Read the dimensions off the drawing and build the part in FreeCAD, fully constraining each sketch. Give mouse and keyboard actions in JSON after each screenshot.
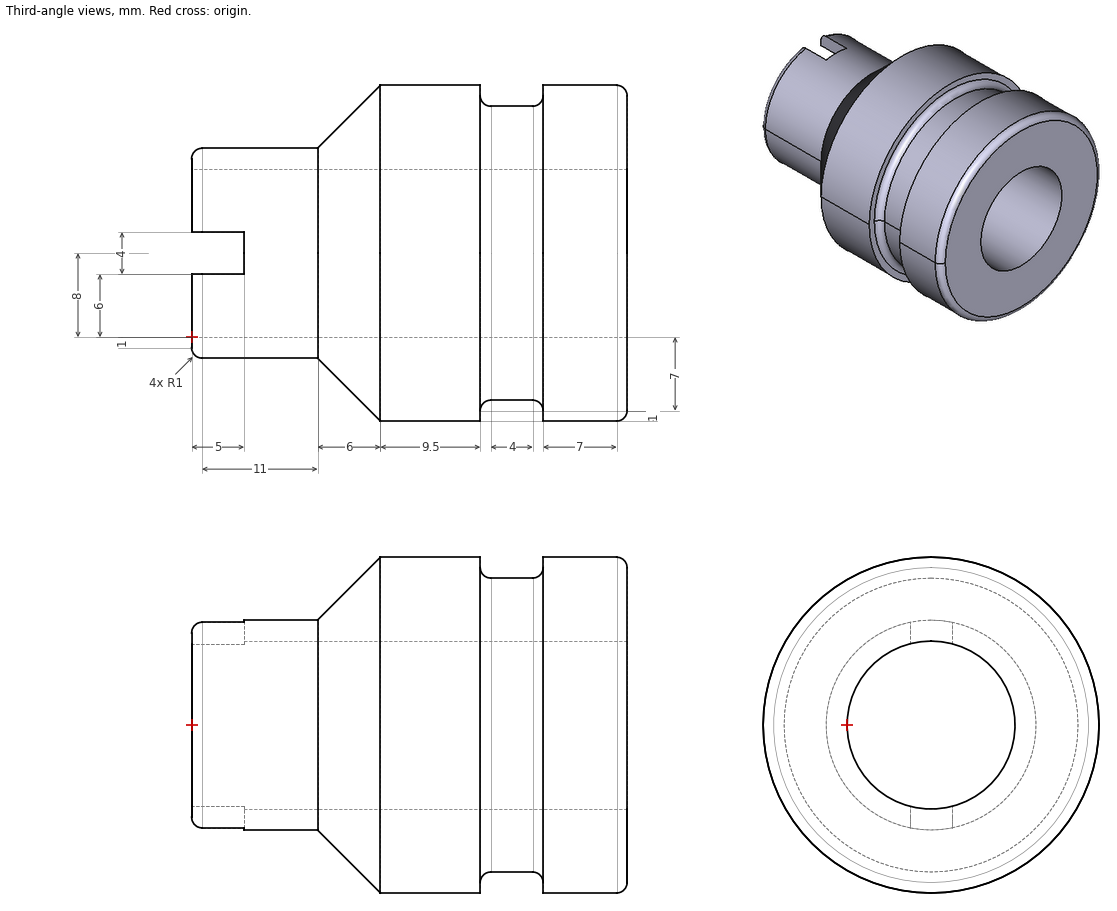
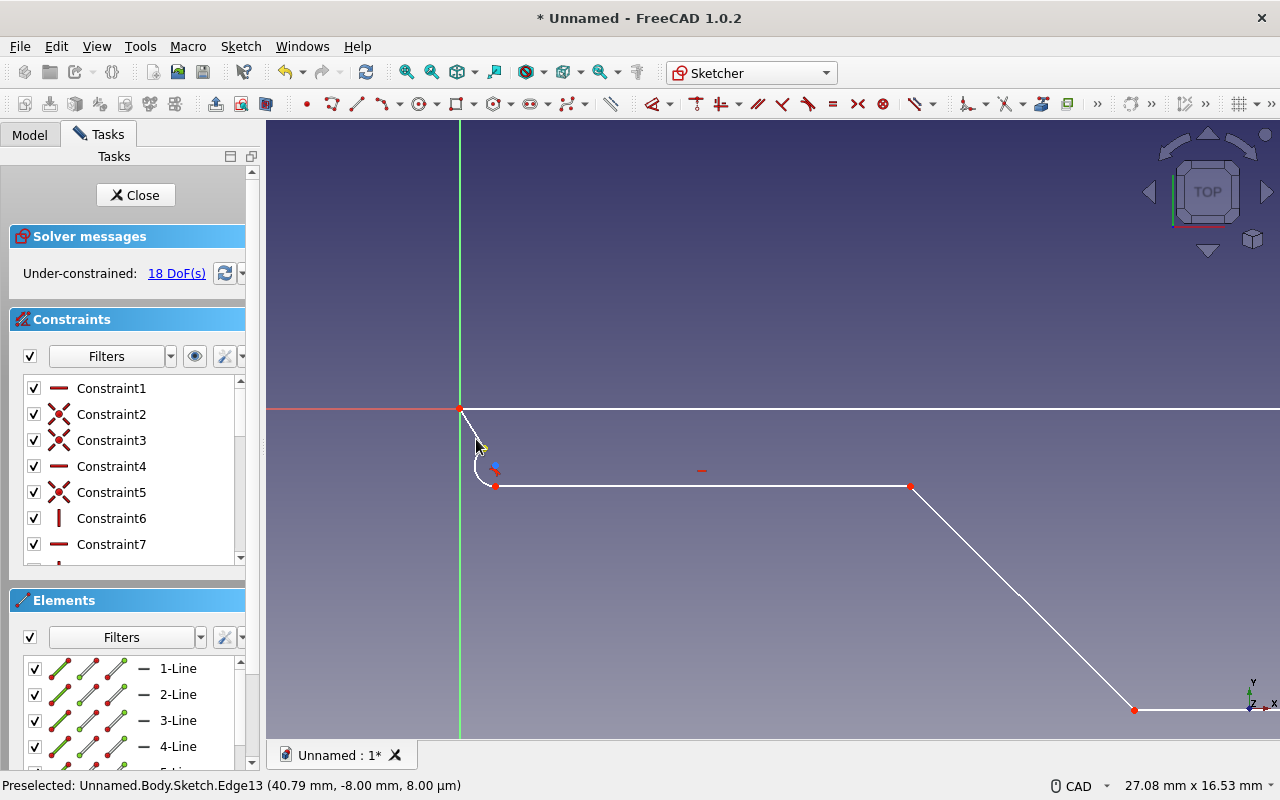
{"action": "left_click", "coordinate": [477, 436]}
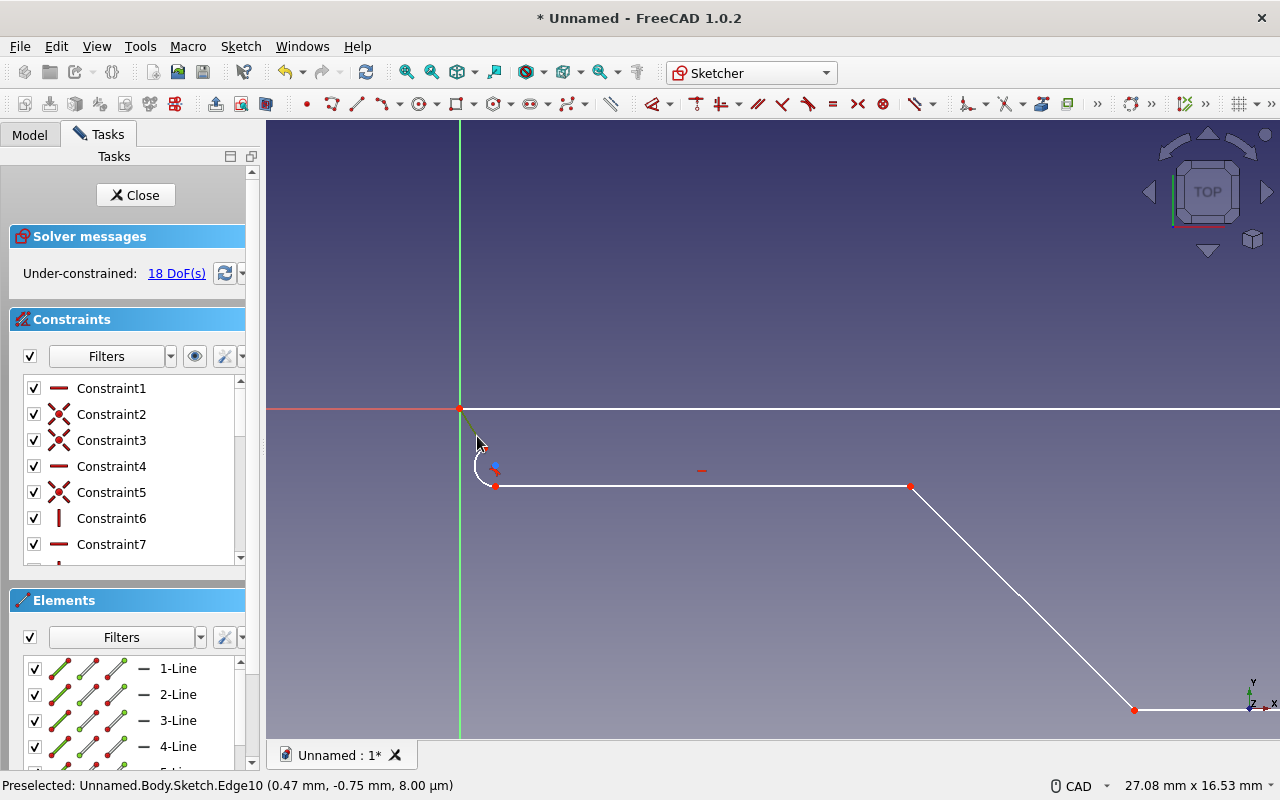
{"action": "left_click", "coordinate": [475, 461]}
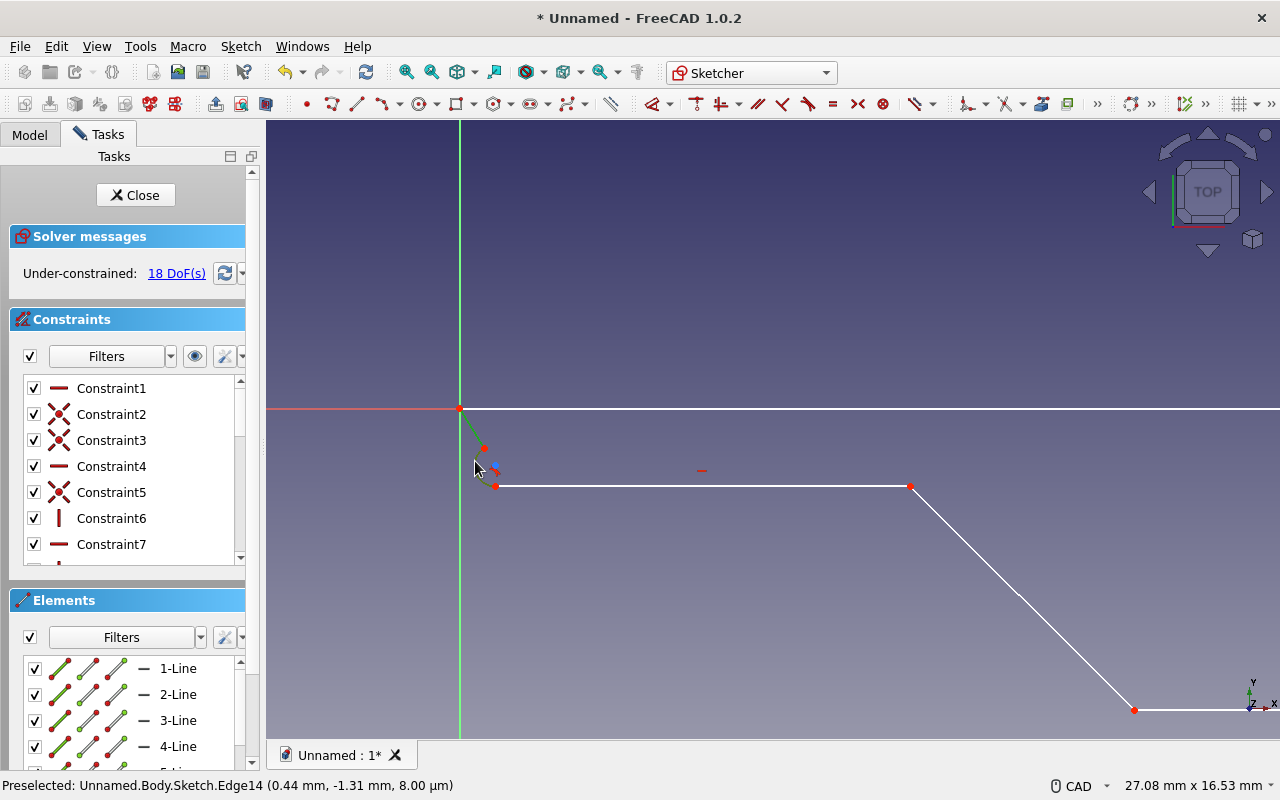
{"action": "key", "text": "t"}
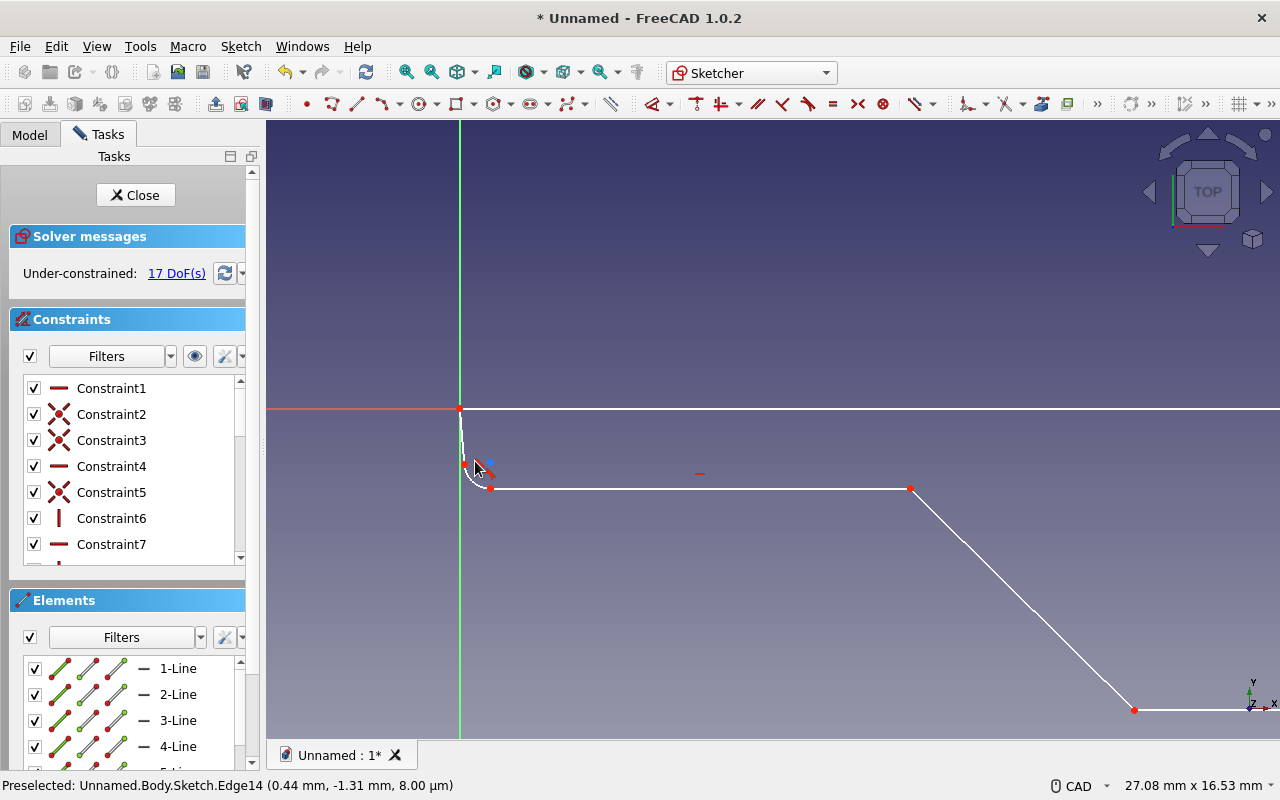
{"action": "left_click", "coordinate": [461, 425]}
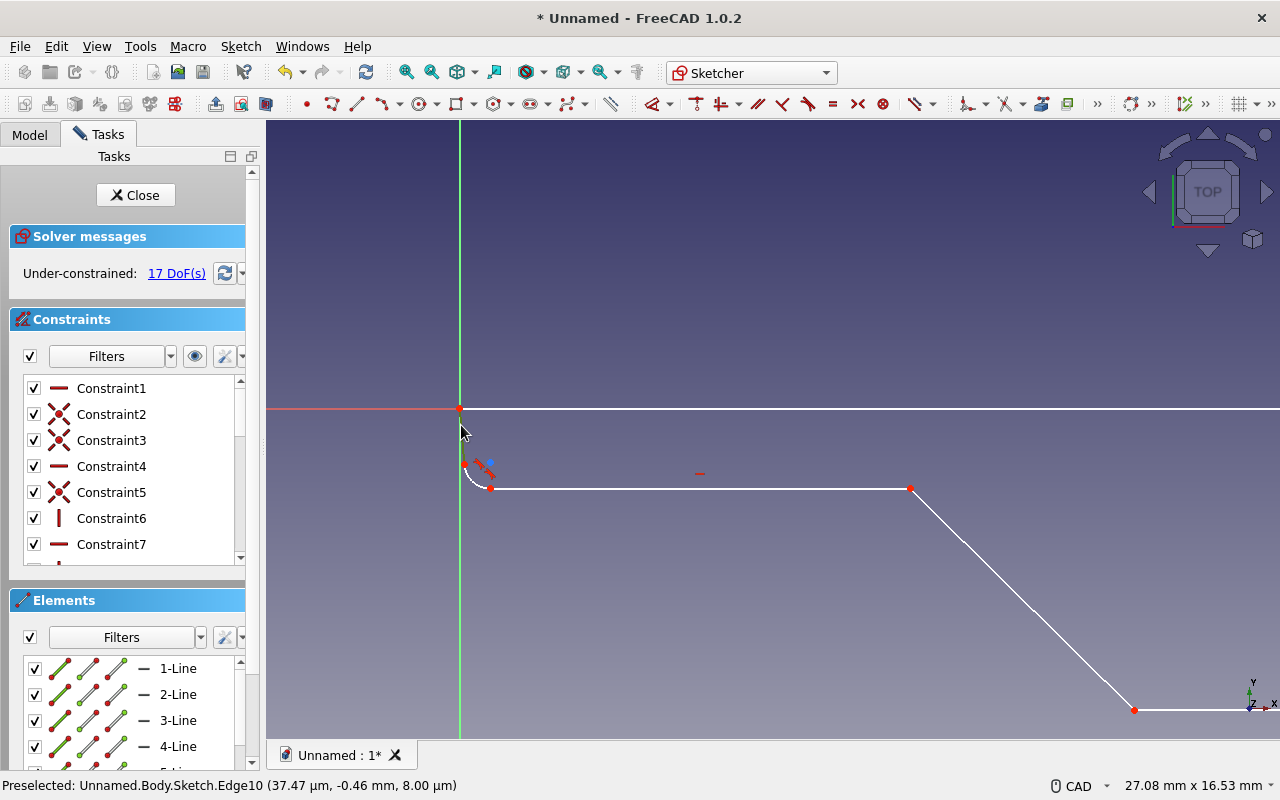
{"action": "key", "text": "v"}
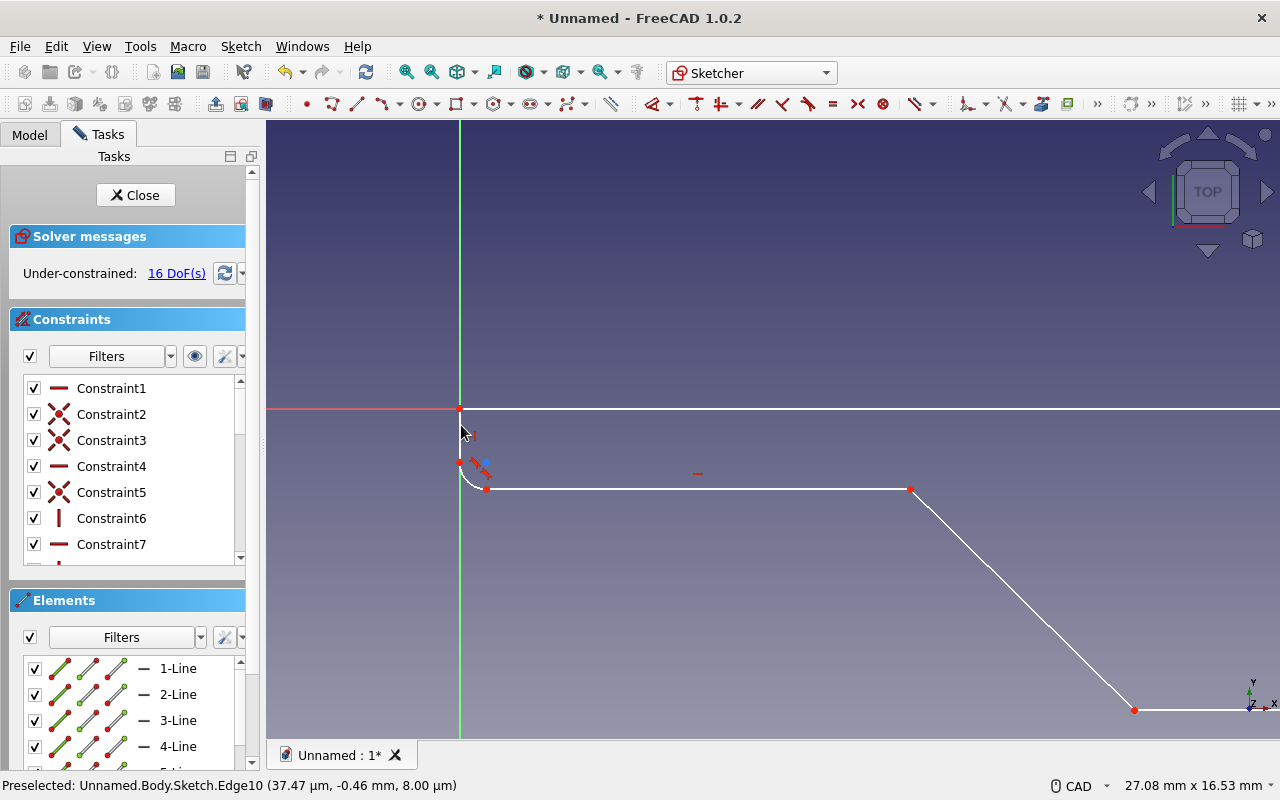
{"action": "scroll", "coordinate": [475, 438], "scroll_direction": "down", "scroll_amount": 6}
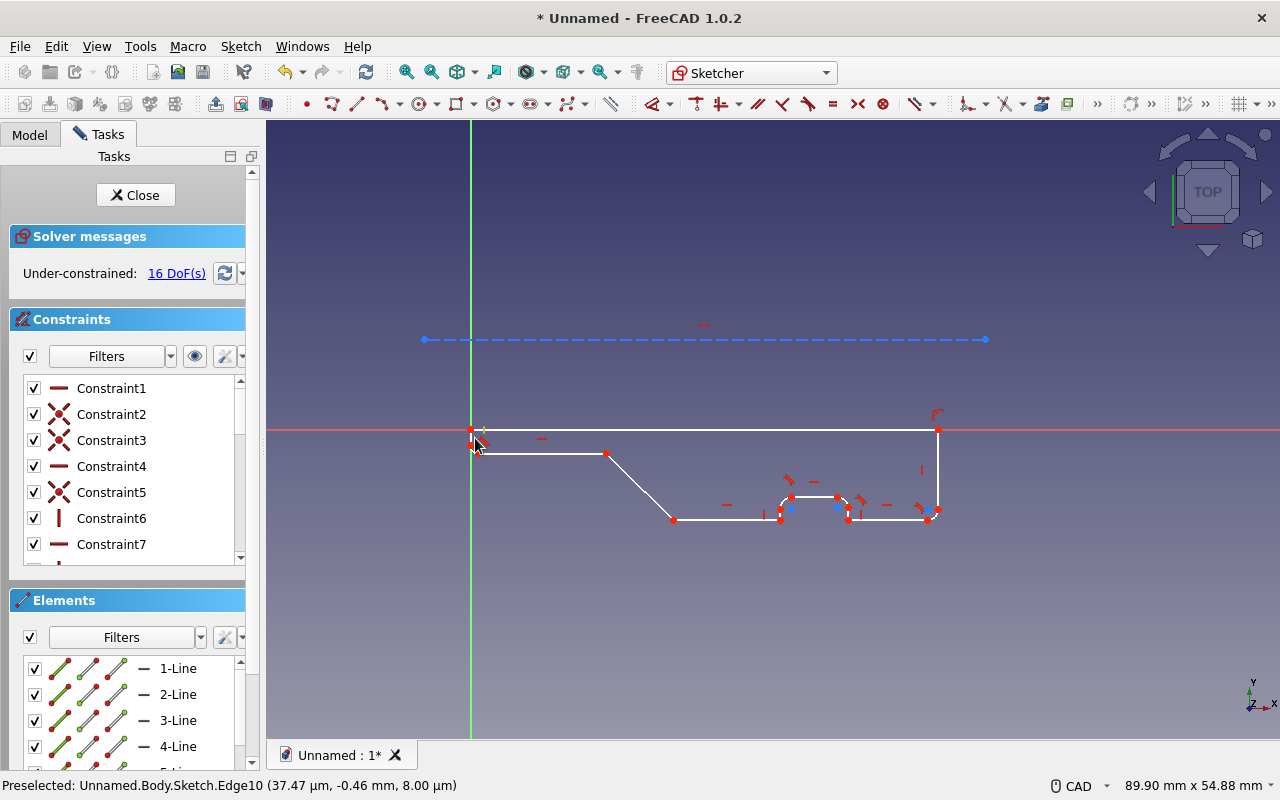
{"action": "scroll", "coordinate": [787, 499], "scroll_direction": "up", "scroll_amount": 5}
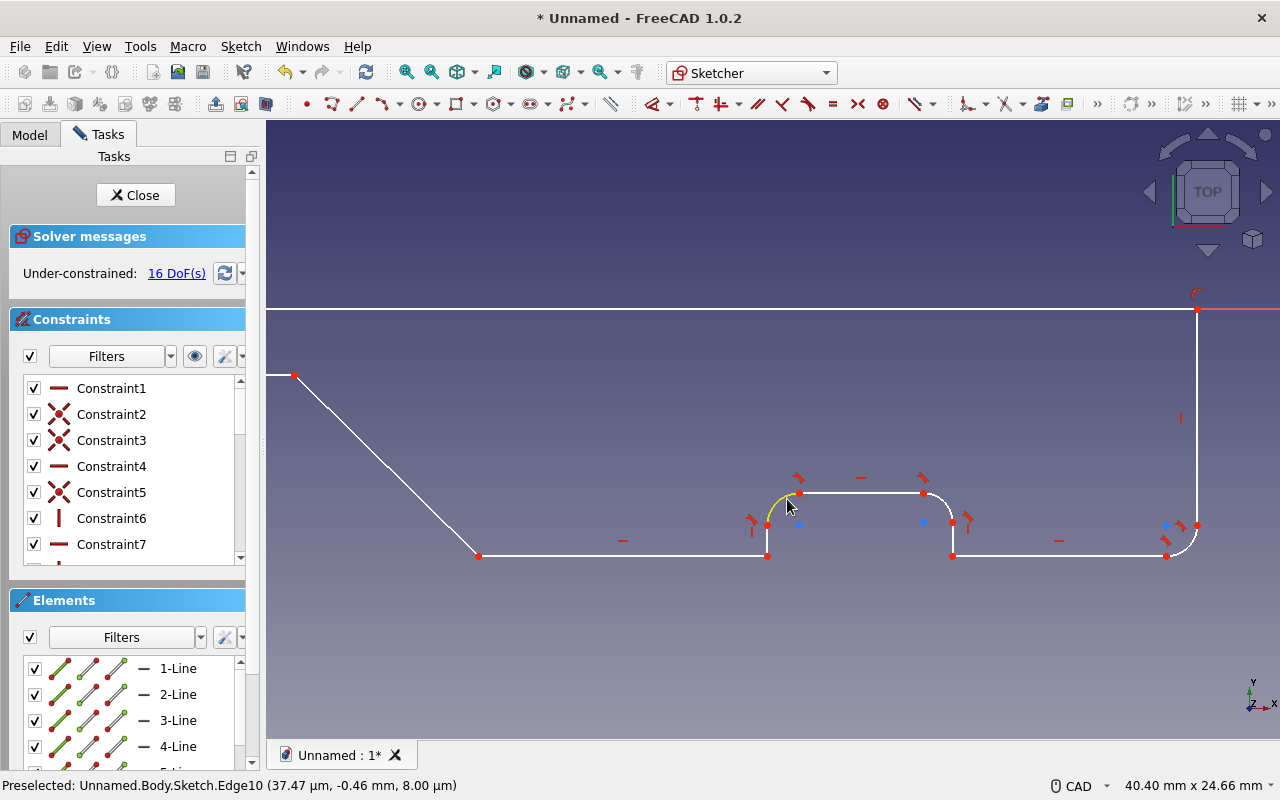
{"action": "left_click", "coordinate": [785, 497]}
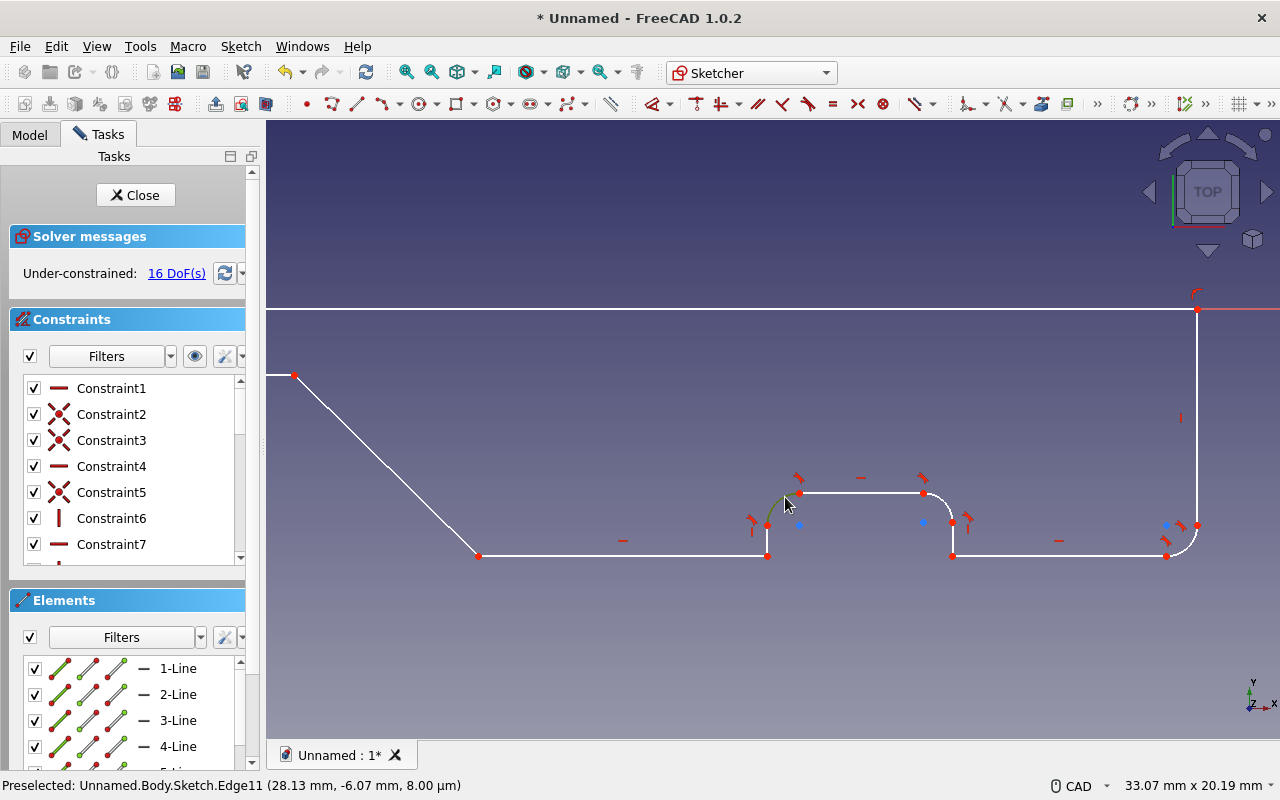
{"action": "left_click", "coordinate": [949, 509]}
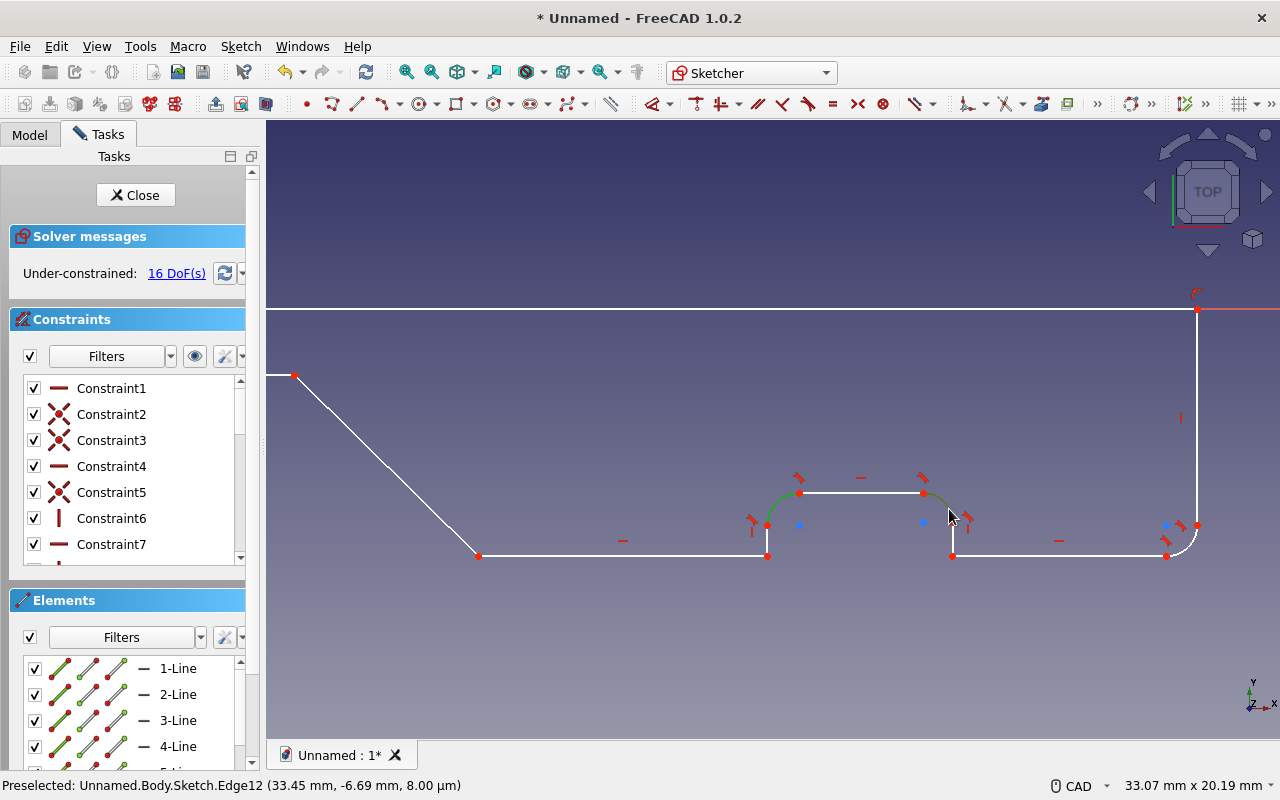
{"action": "scroll", "coordinate": [787, 500], "scroll_direction": "down", "scroll_amount": 5}